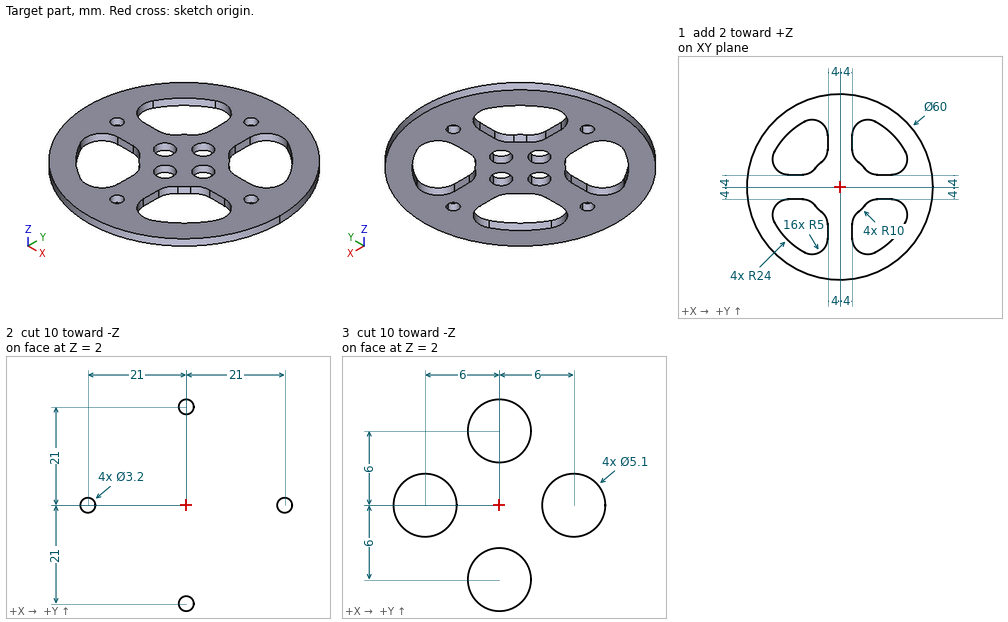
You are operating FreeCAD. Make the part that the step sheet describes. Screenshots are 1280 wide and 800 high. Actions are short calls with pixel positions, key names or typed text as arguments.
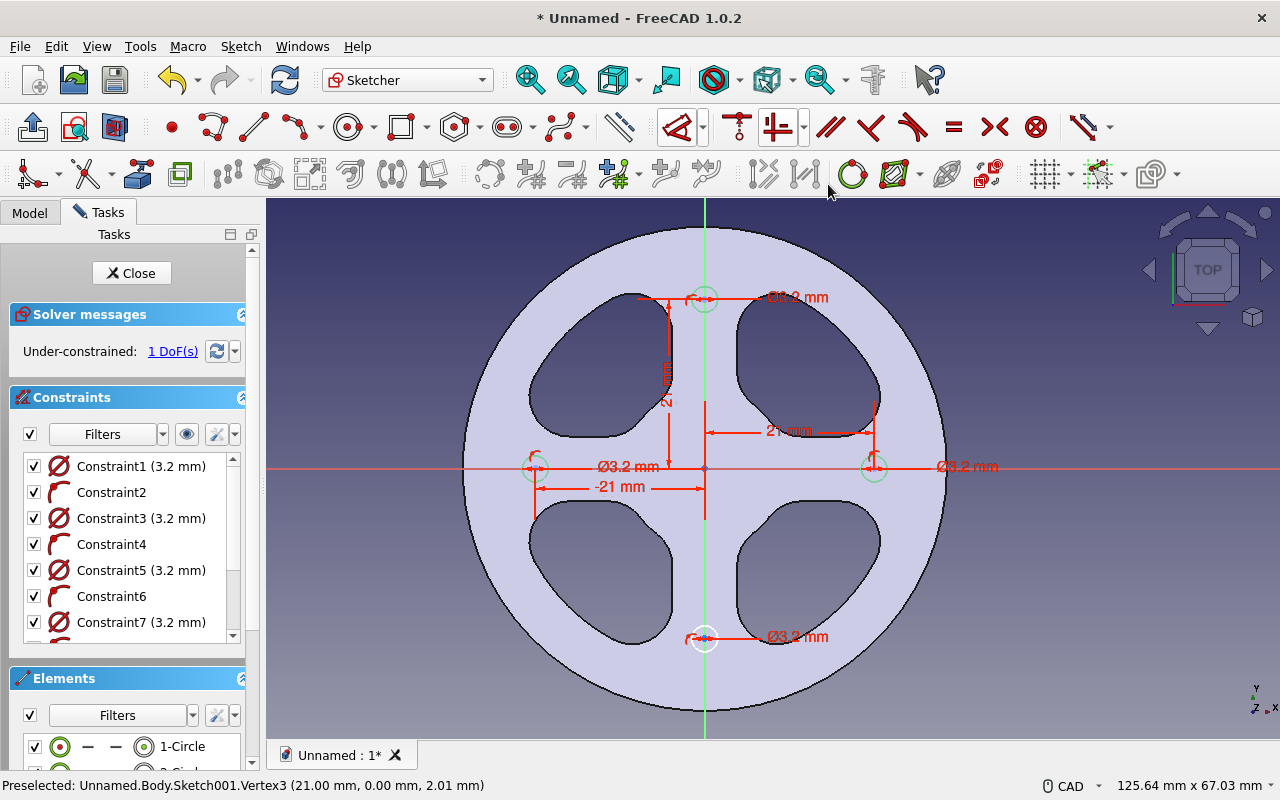
click(705, 639)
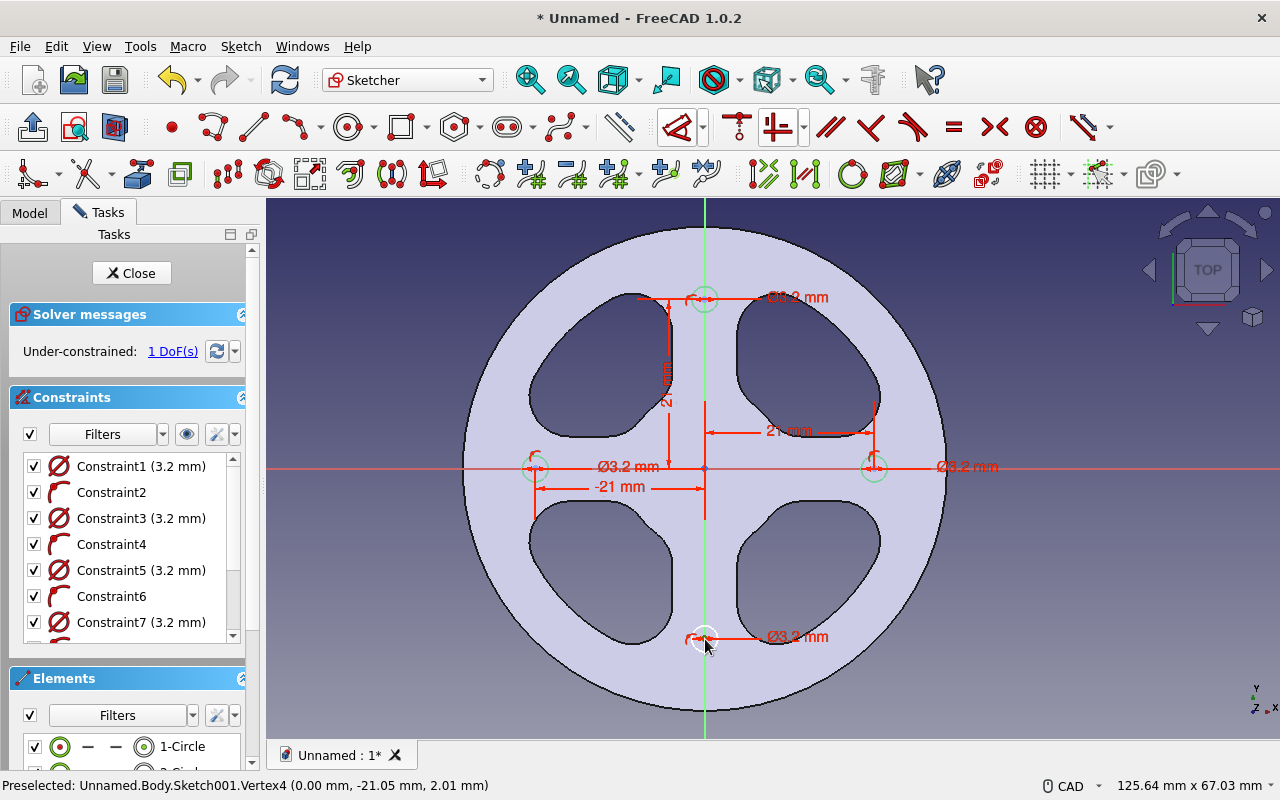
click(702, 128)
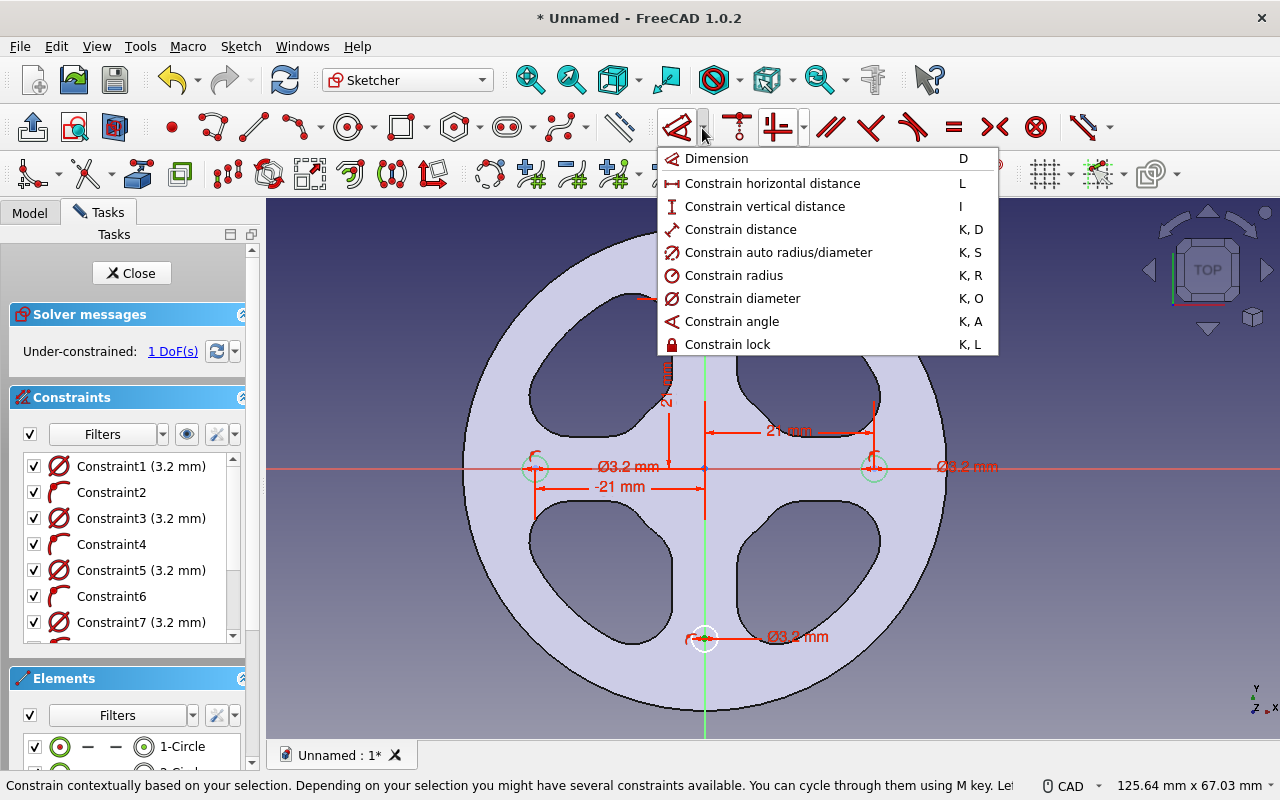
click(828, 206)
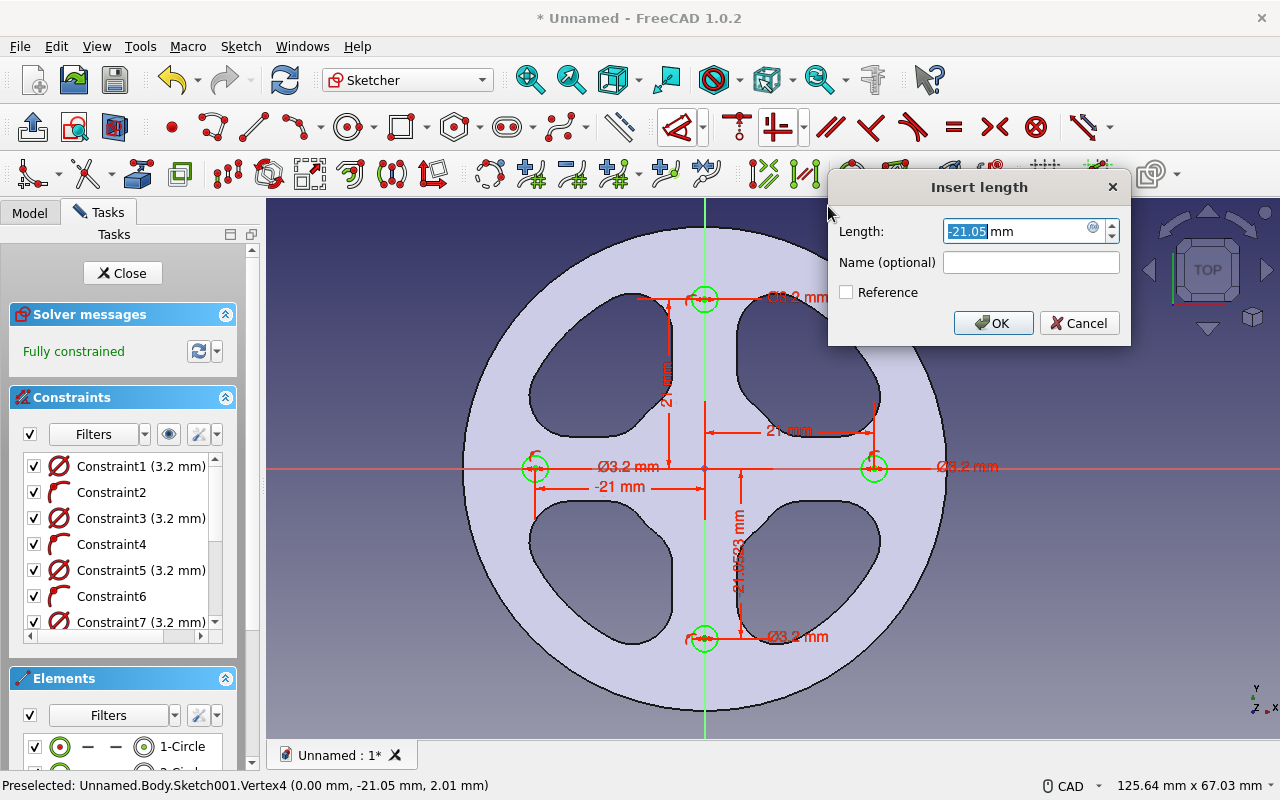
text(-21)
key(Return)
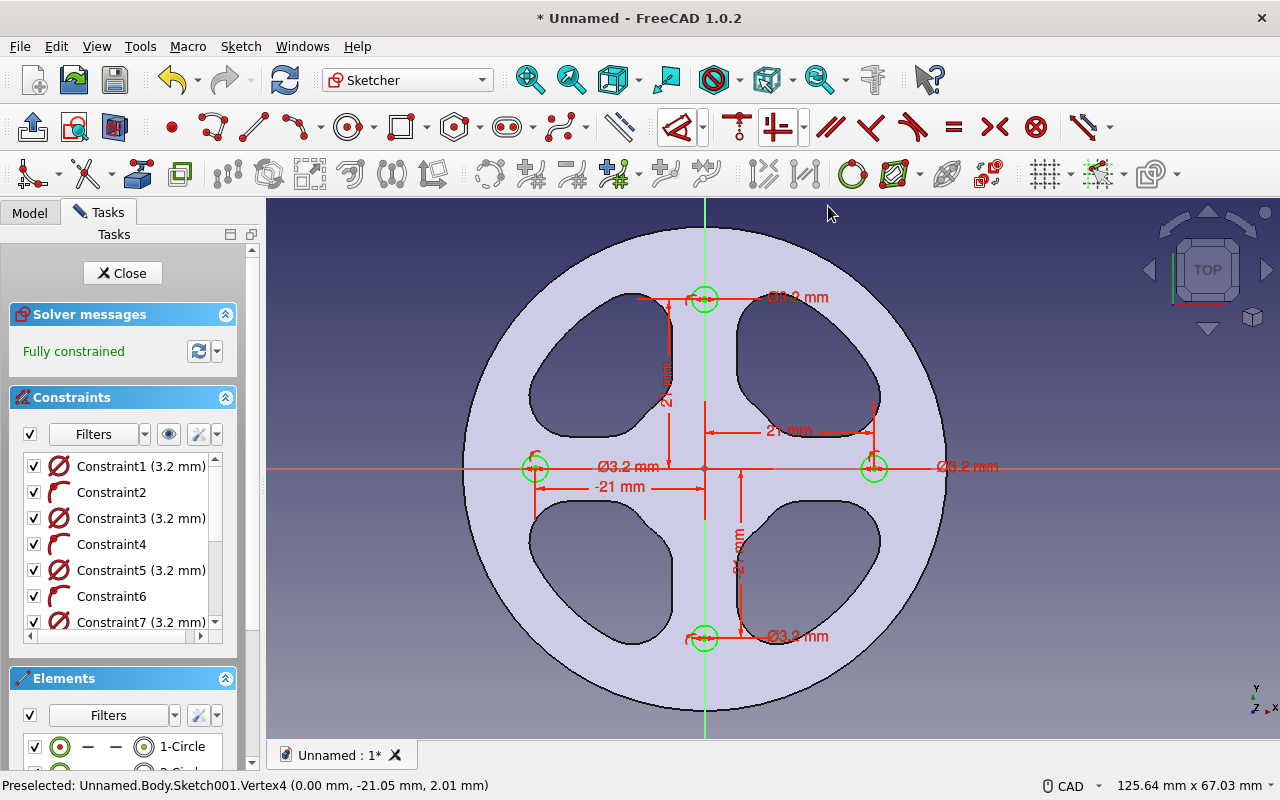
click(123, 273)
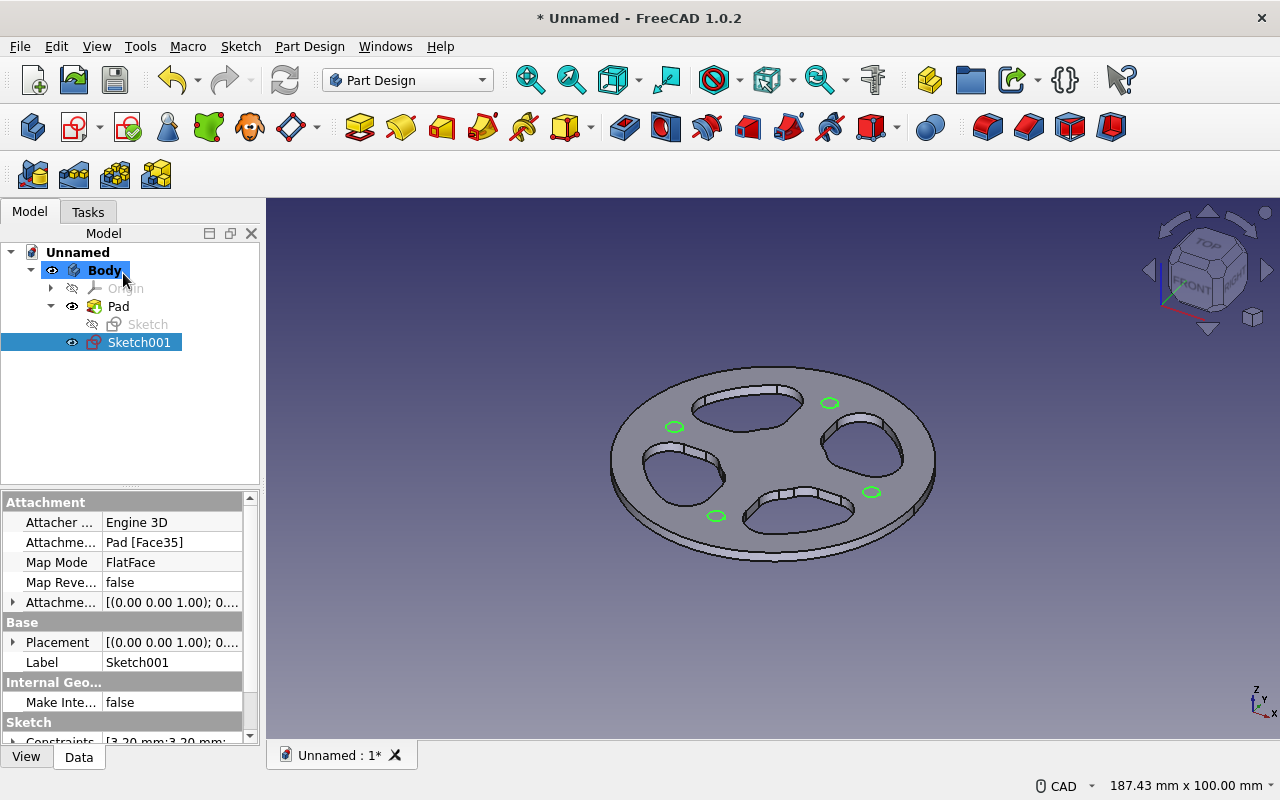
click(625, 128)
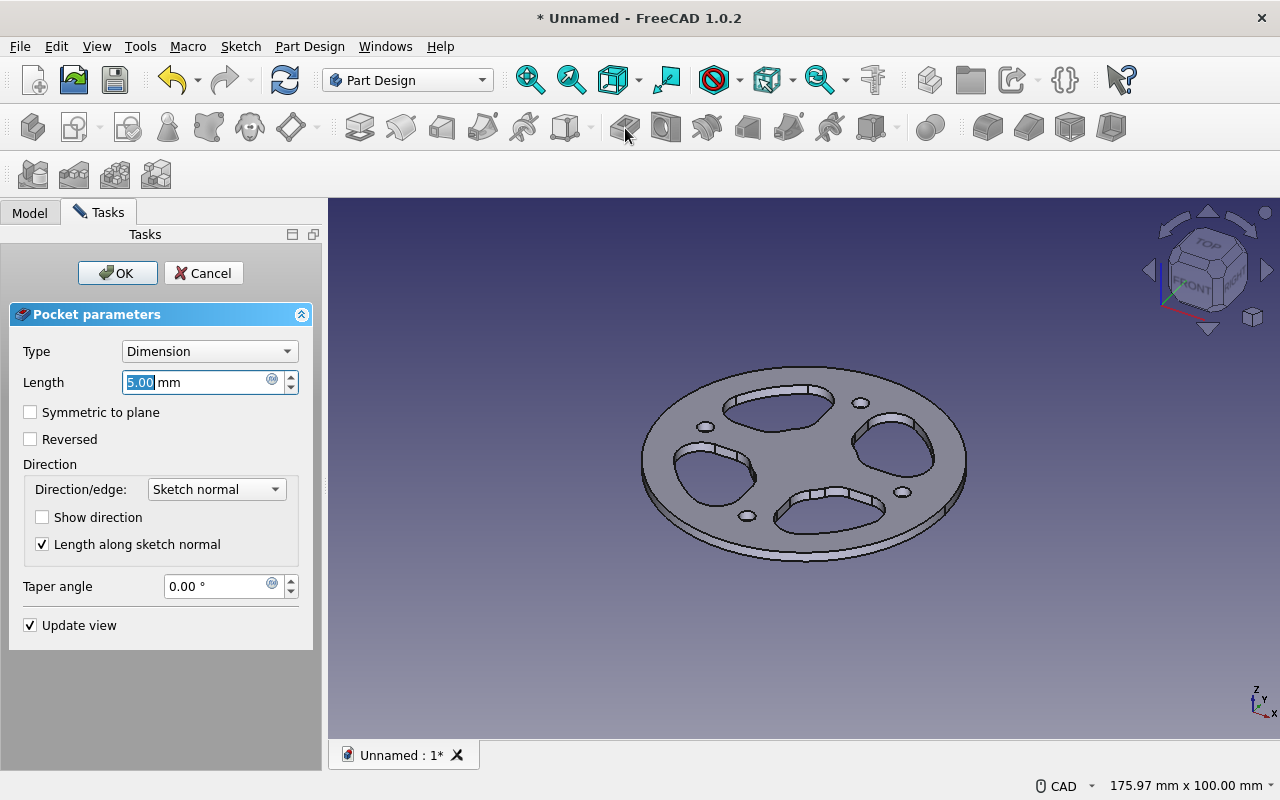
text(10)
key(Tab)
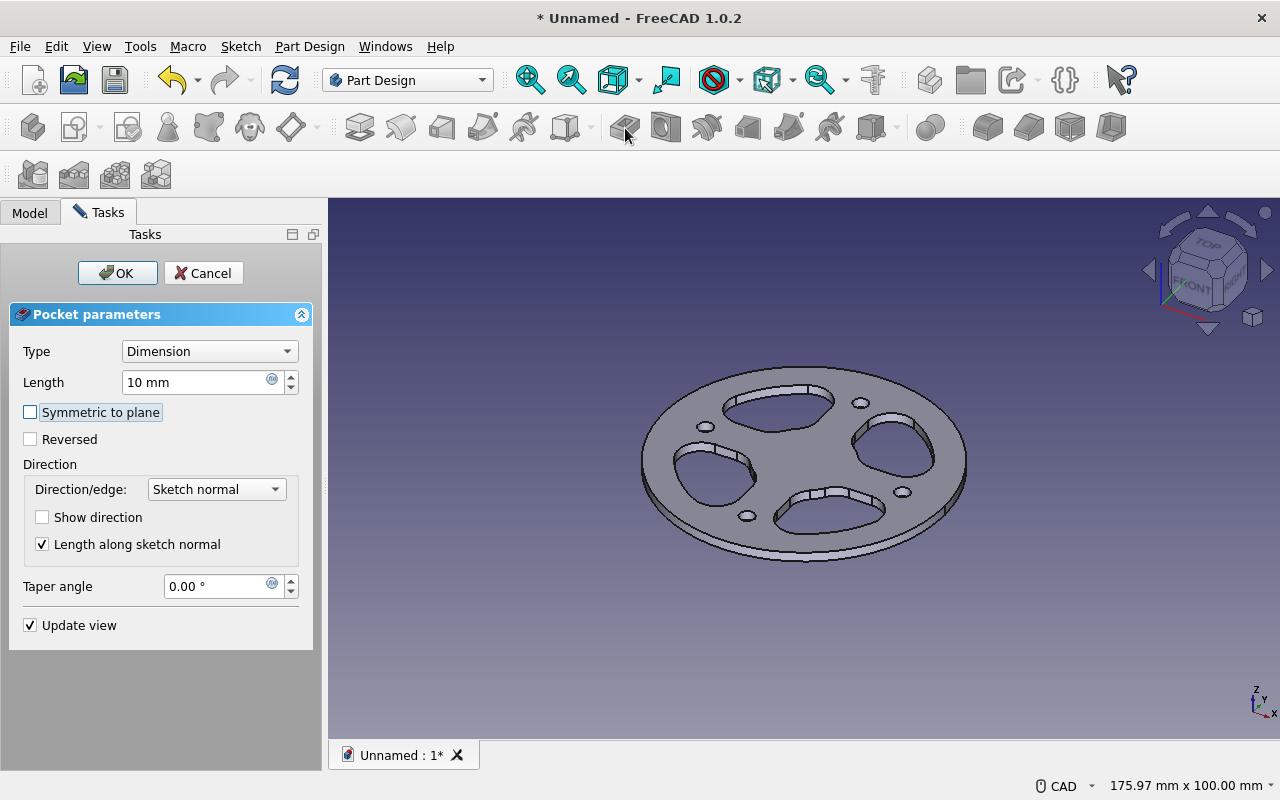
click(118, 273)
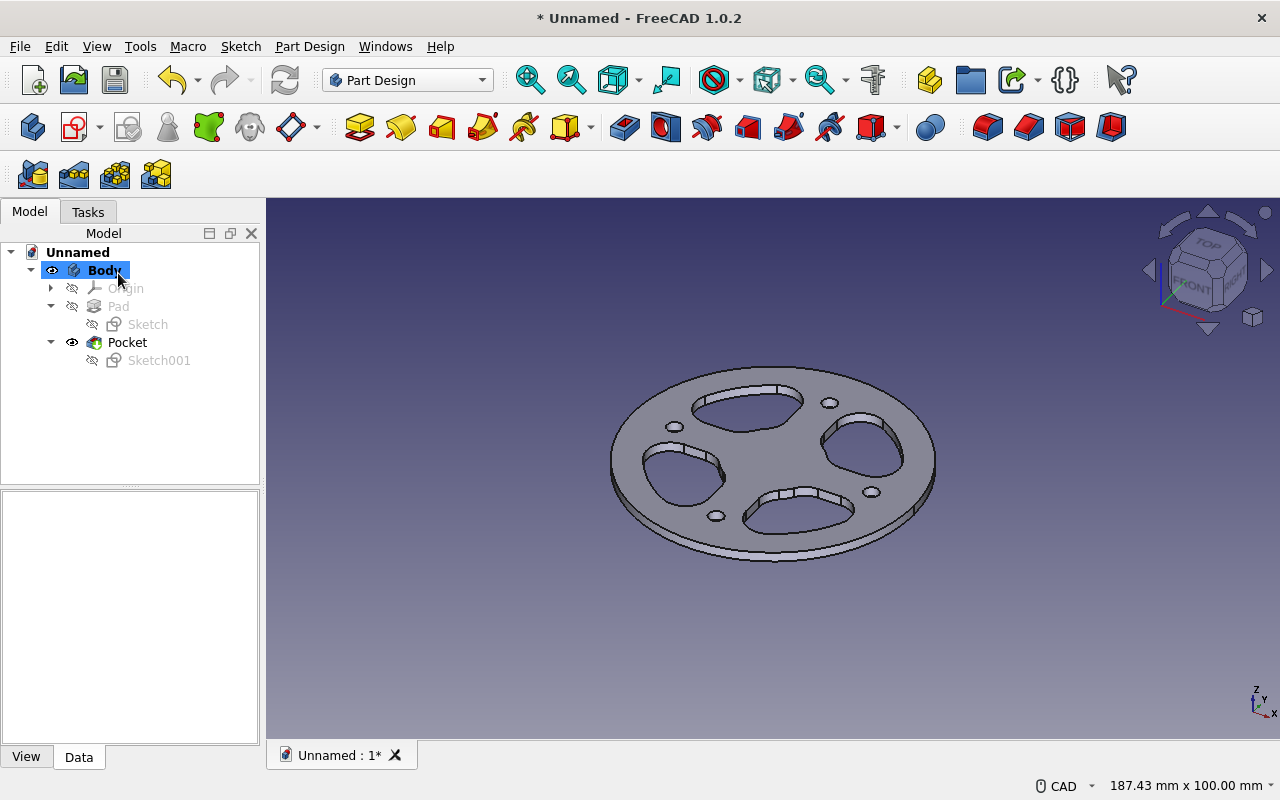
click(773, 459)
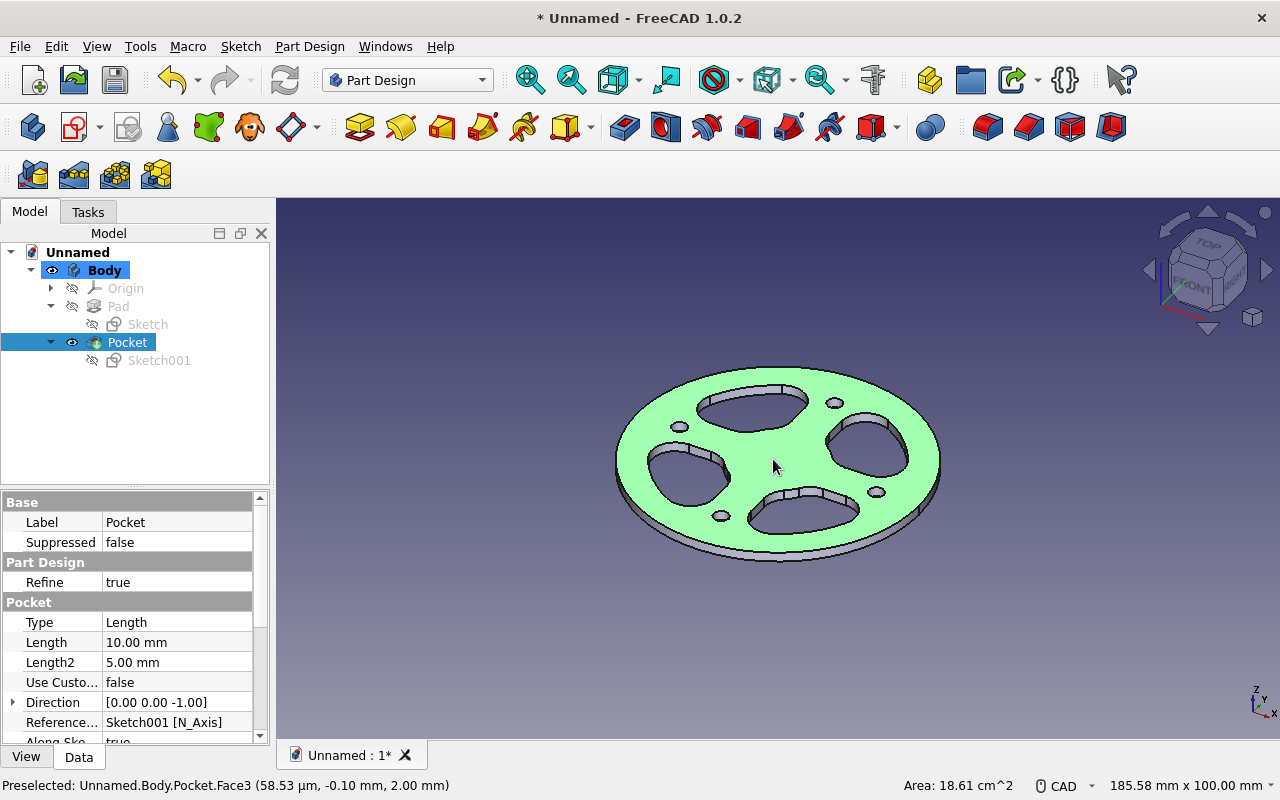
click(74, 128)